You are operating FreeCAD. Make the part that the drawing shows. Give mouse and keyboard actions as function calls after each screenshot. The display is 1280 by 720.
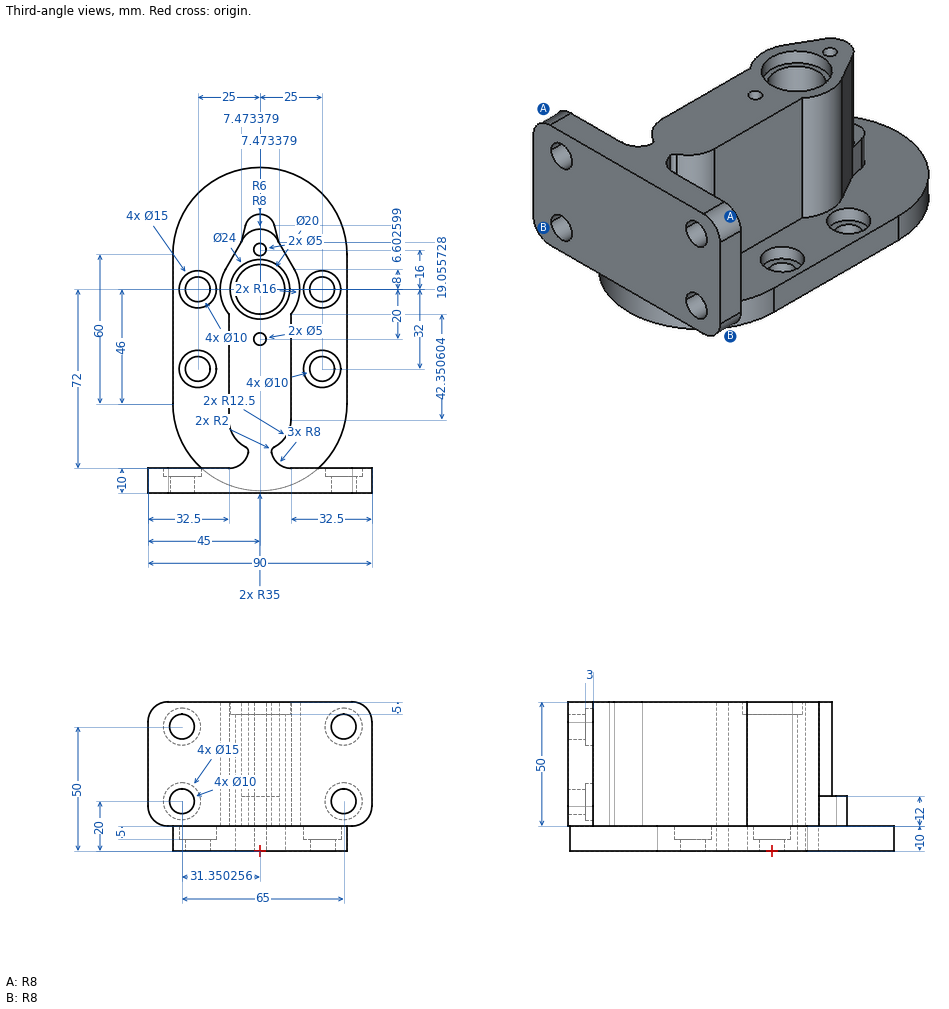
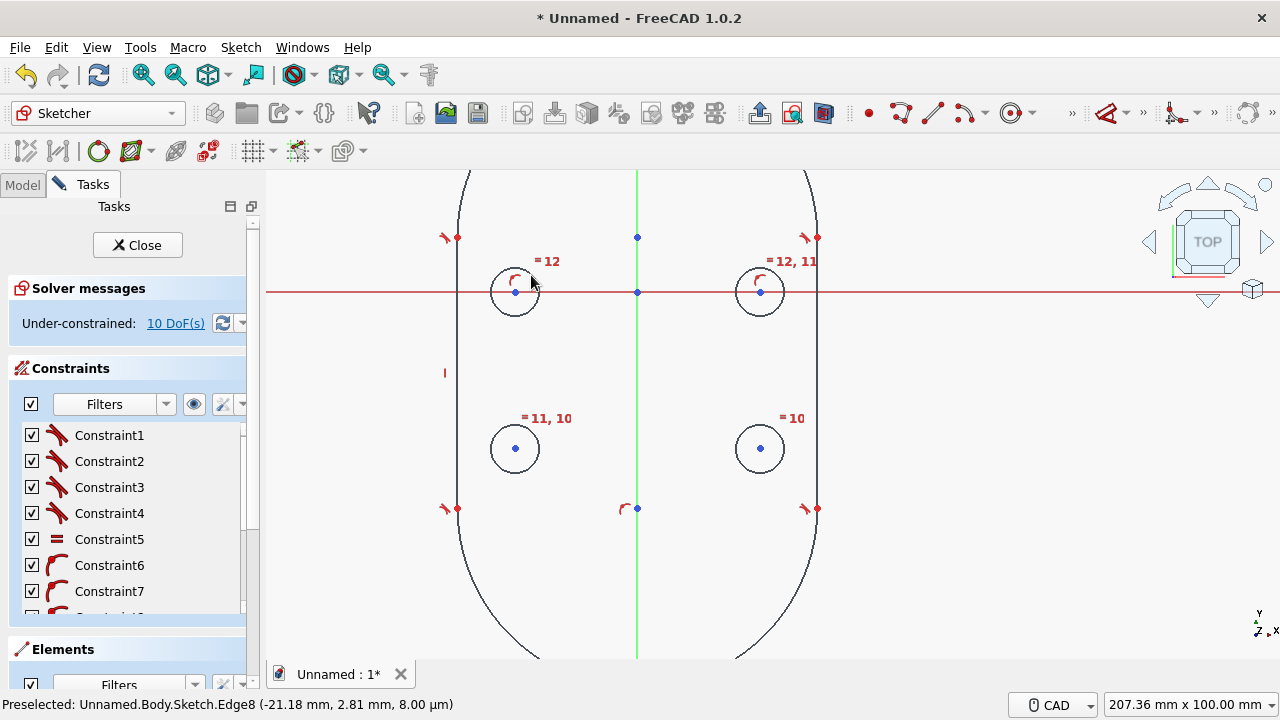
click(1106, 114)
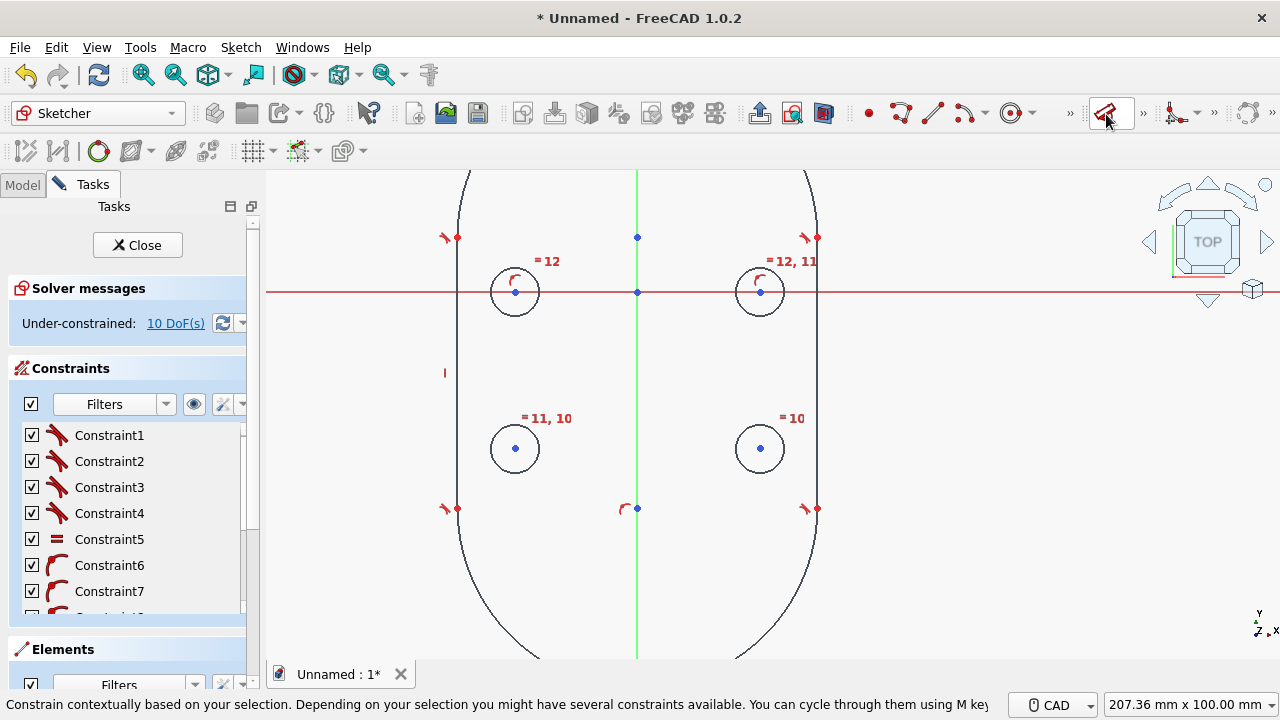
click(492, 614)
click(427, 535)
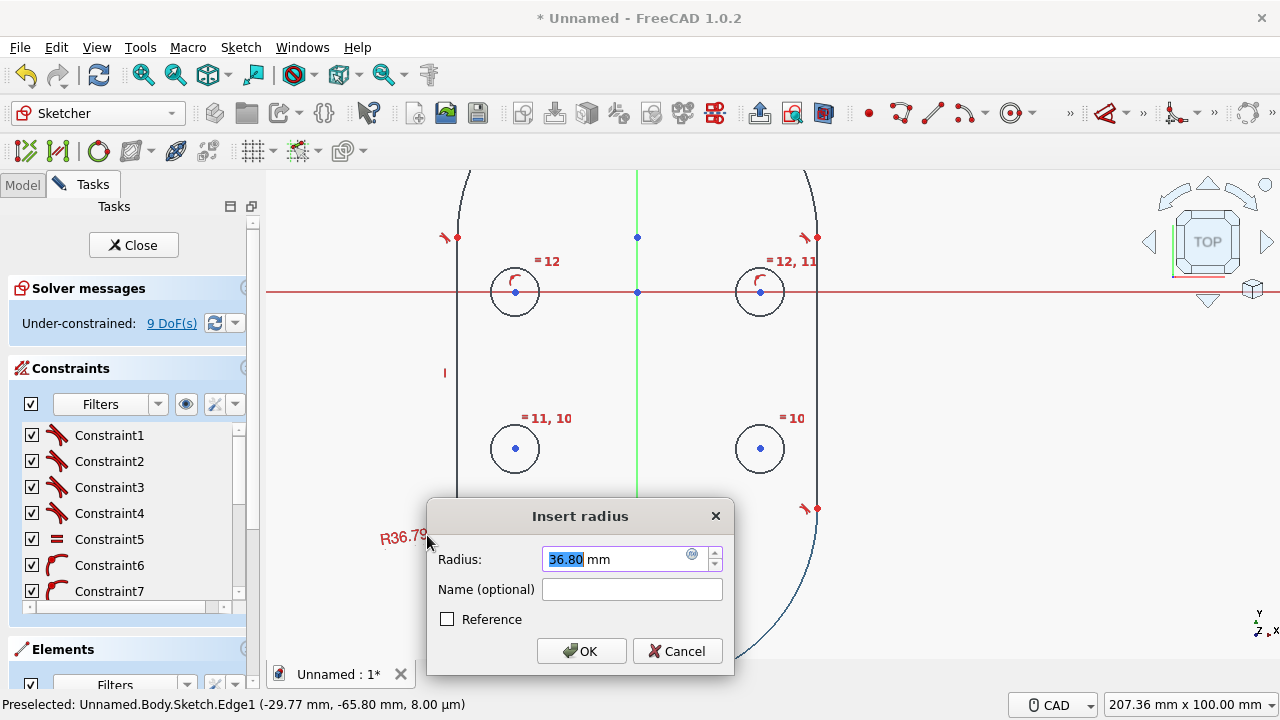
text(35)
key(Return)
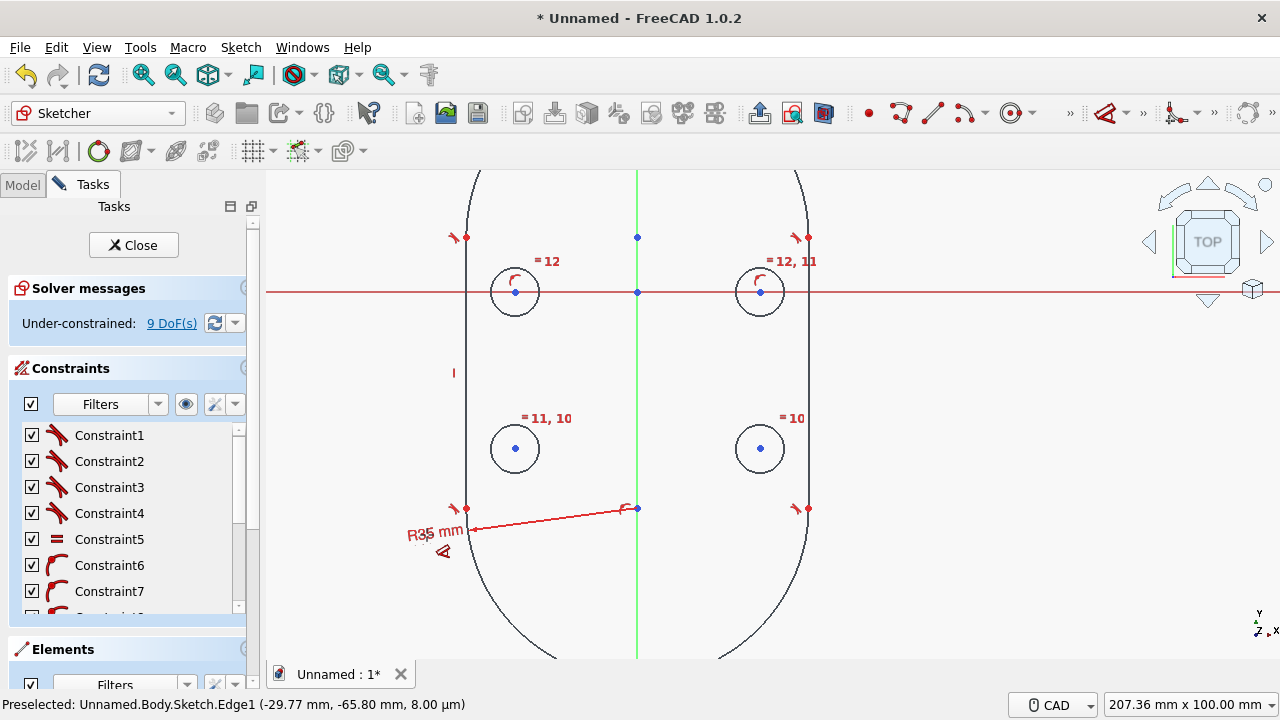
click(777, 432)
click(776, 395)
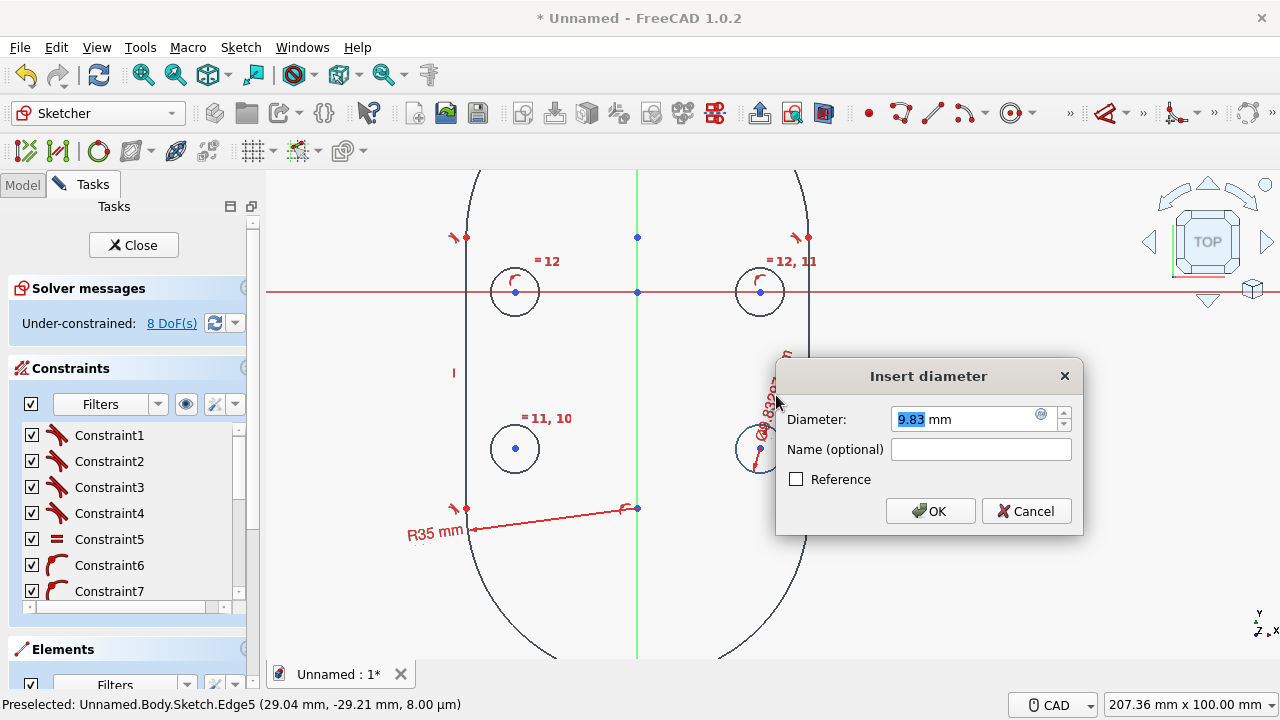
text(10)
key(Return)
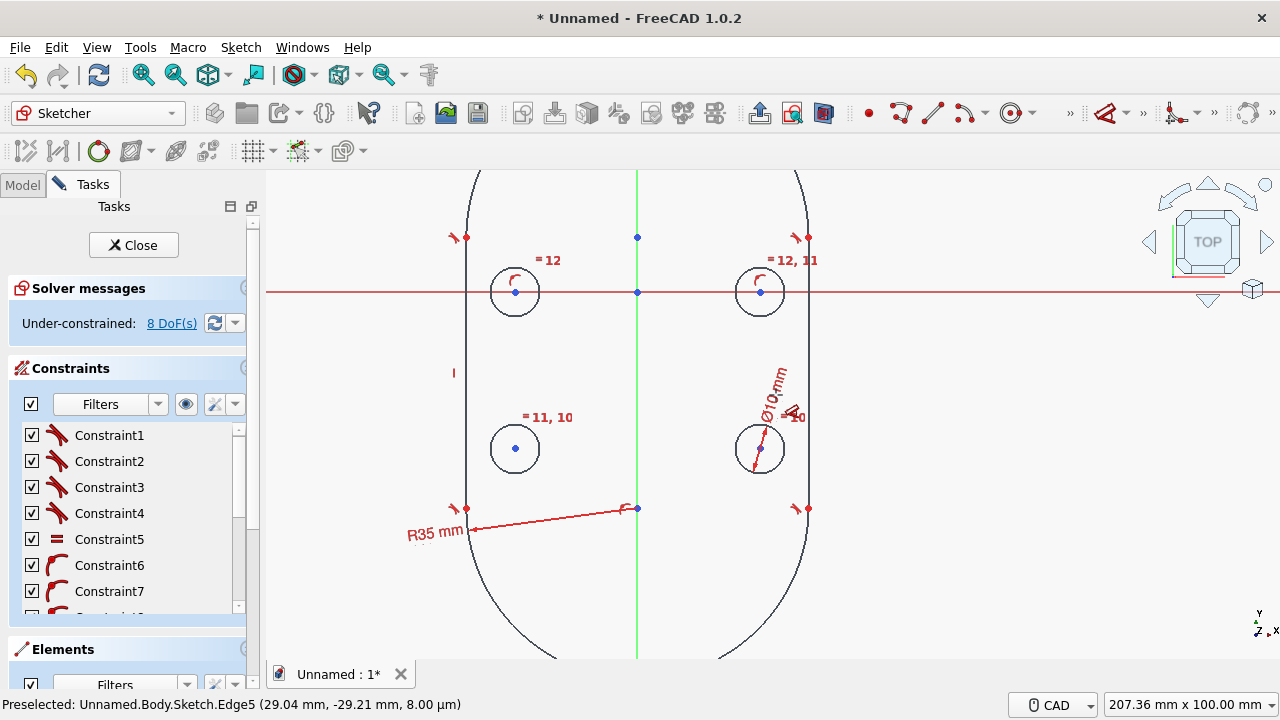
click(466, 427)
click(432, 373)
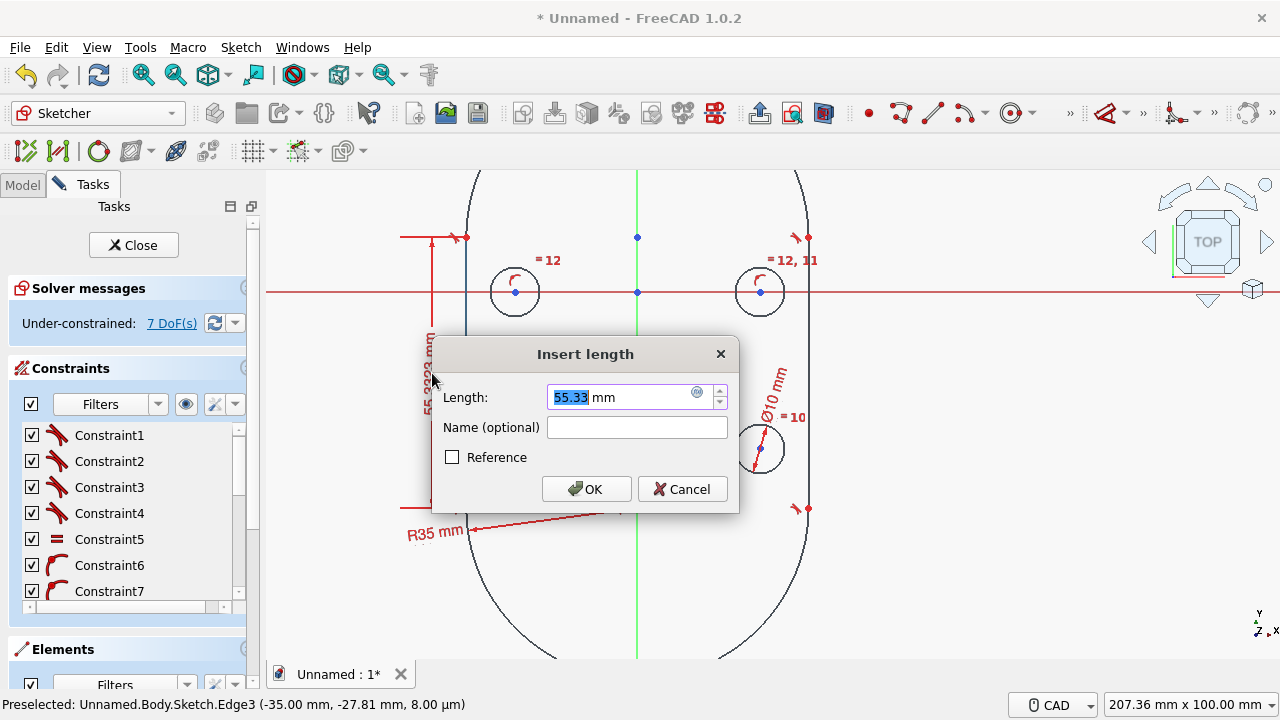
text(60)
key(Return)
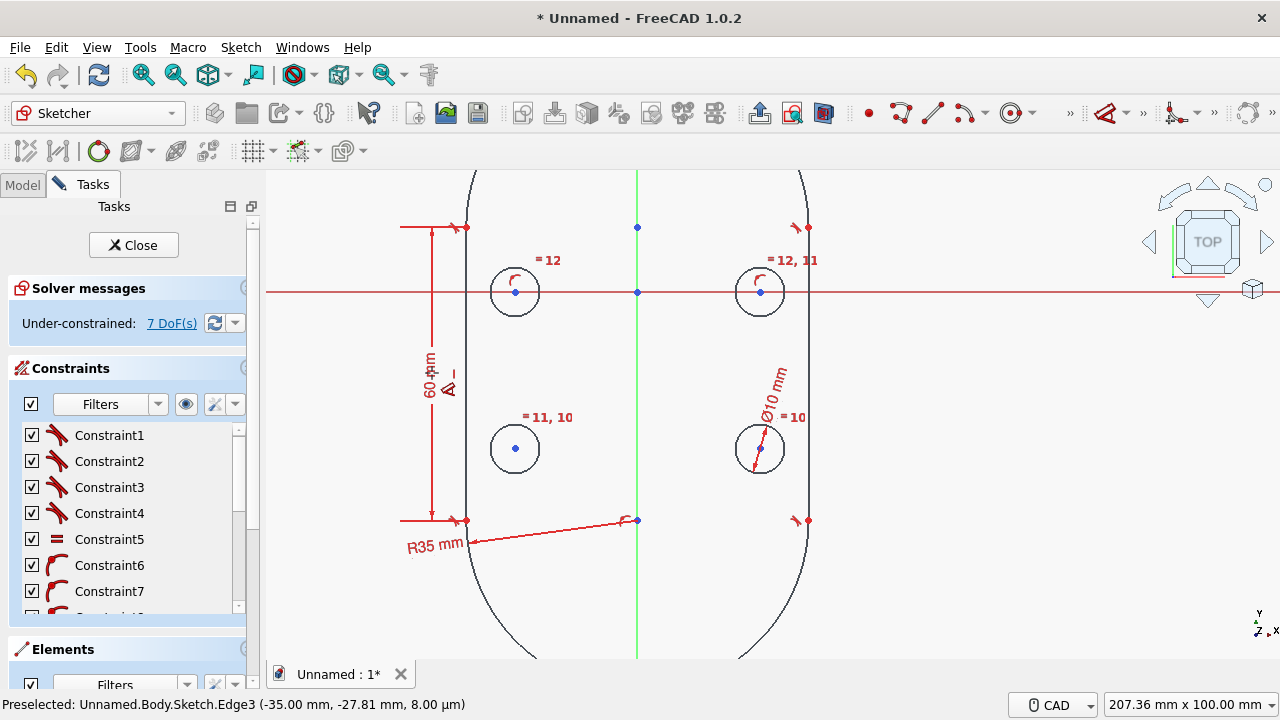
click(760, 449)
click(699, 483)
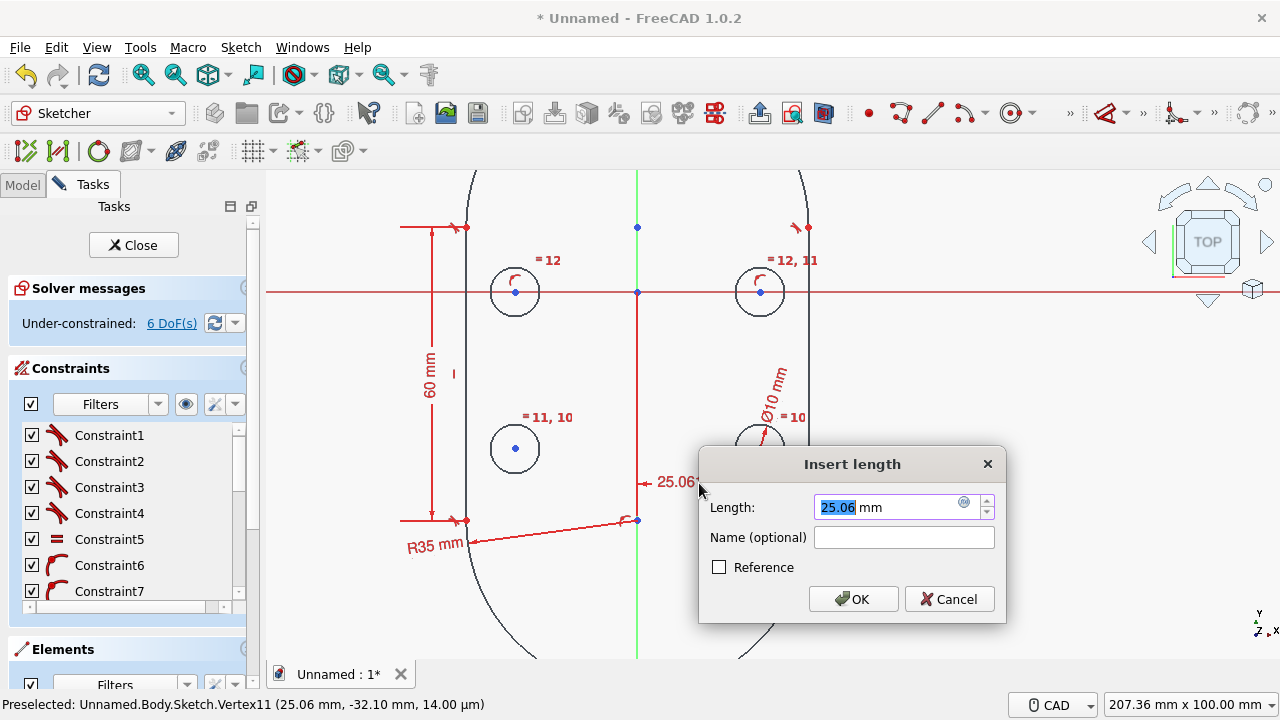
text(25)
key(Return)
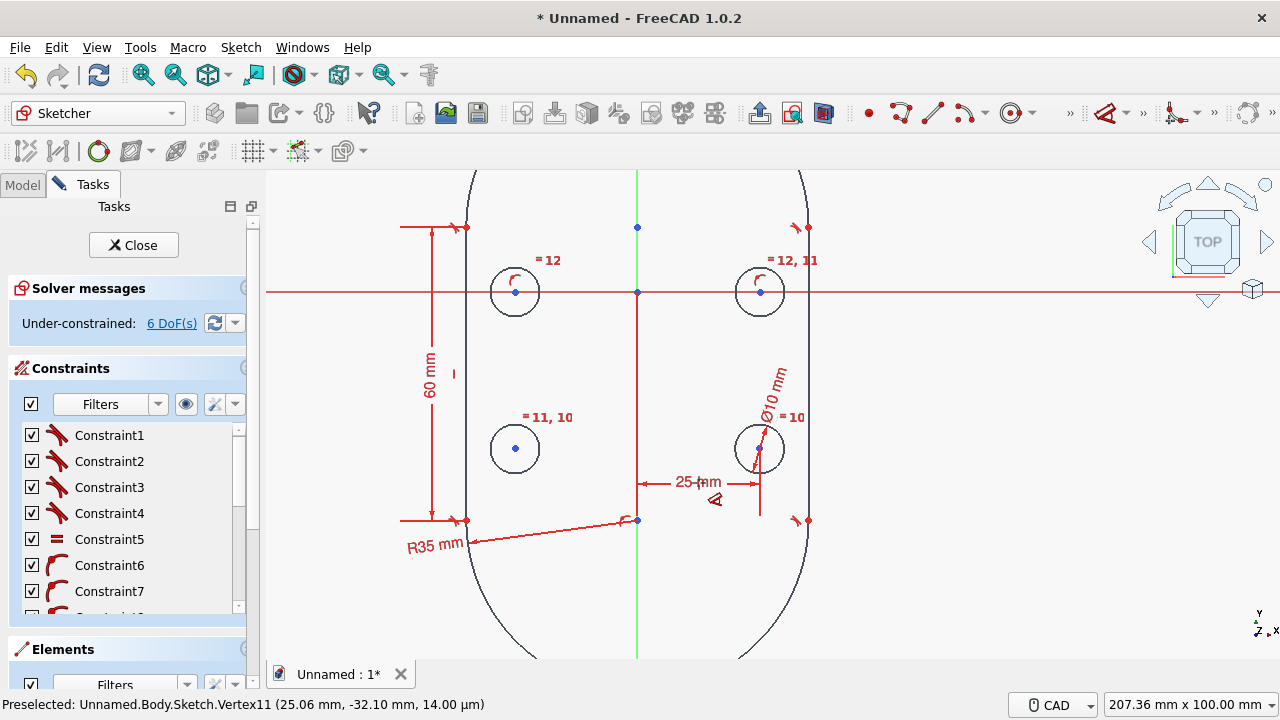
click(760, 449)
click(794, 371)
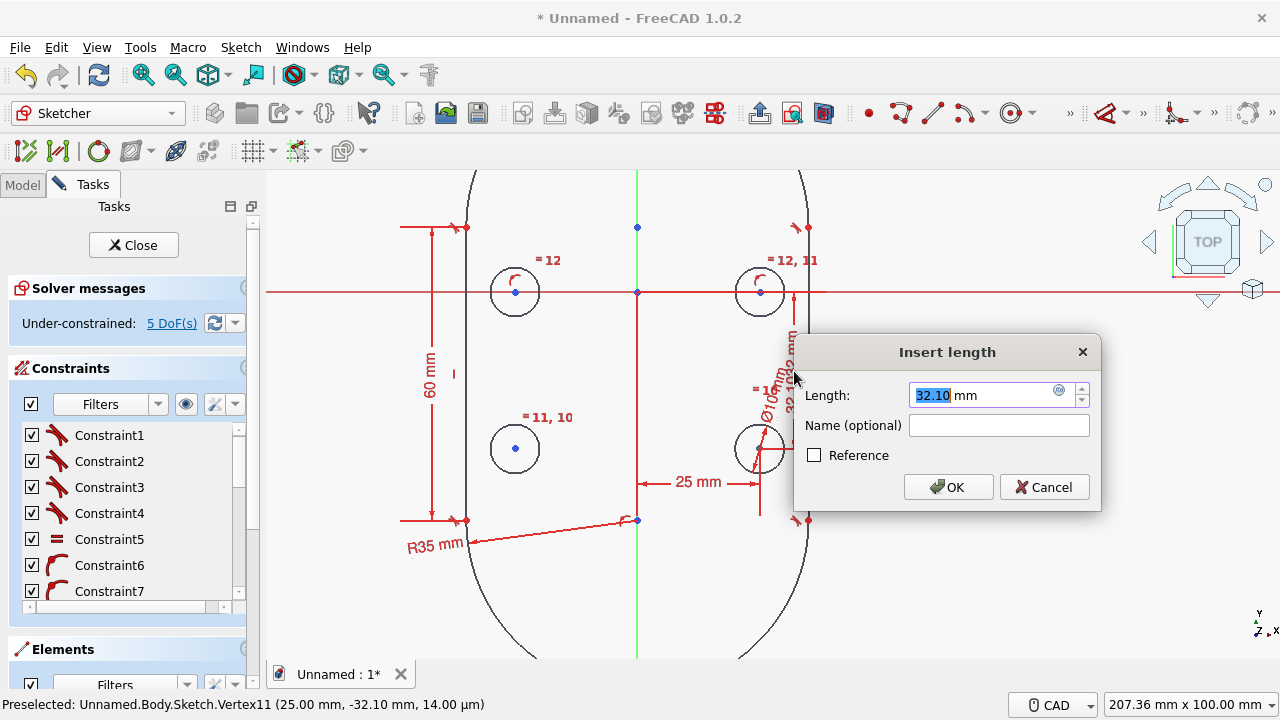
text(32)
key(Return)